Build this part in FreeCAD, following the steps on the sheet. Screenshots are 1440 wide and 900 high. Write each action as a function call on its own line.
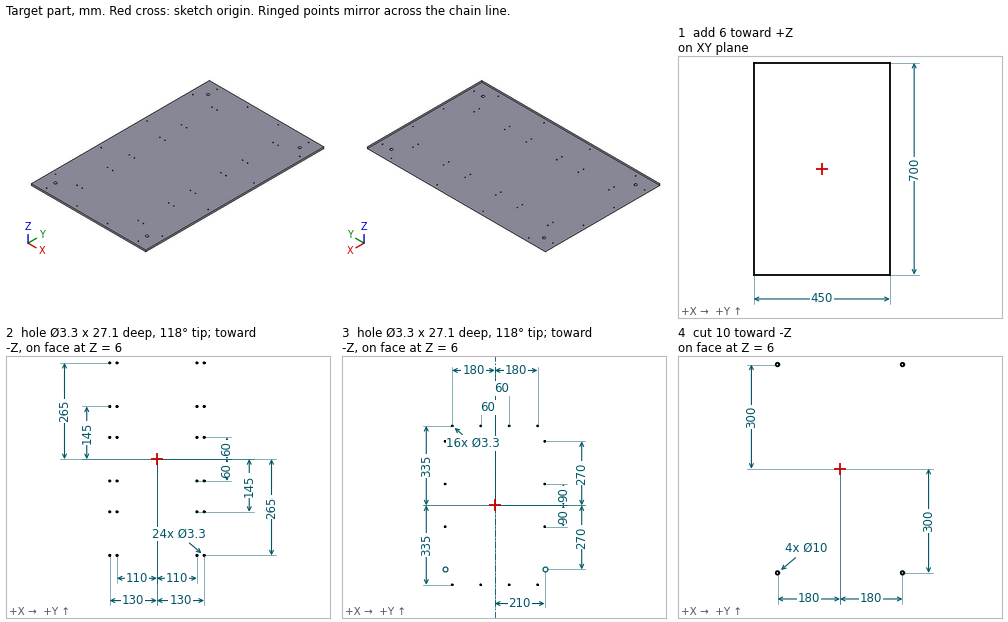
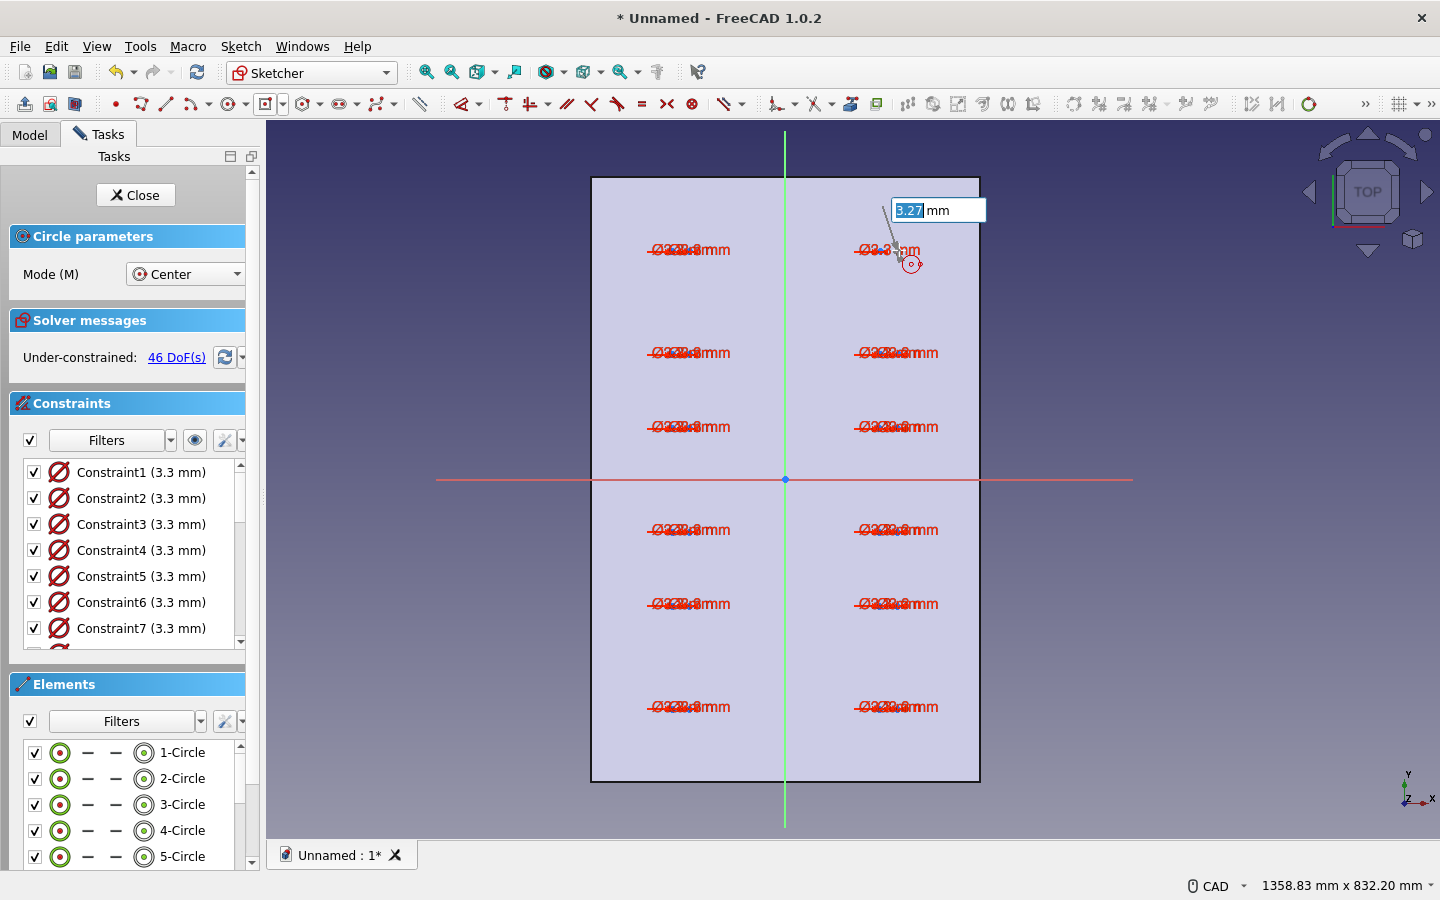
text(3.3)
key(Return)
key(Escape)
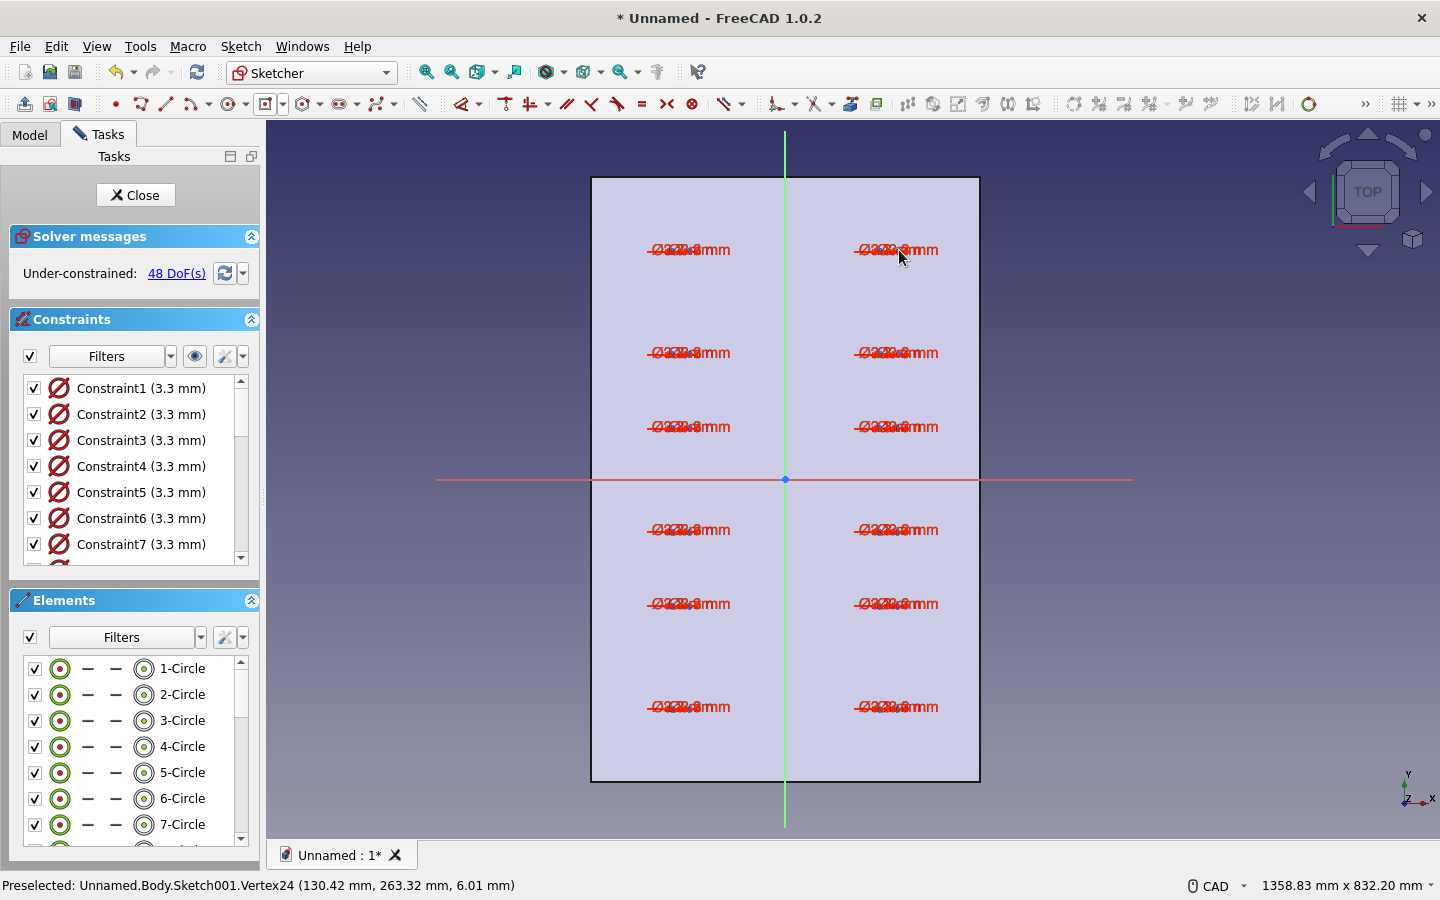
click(898, 709)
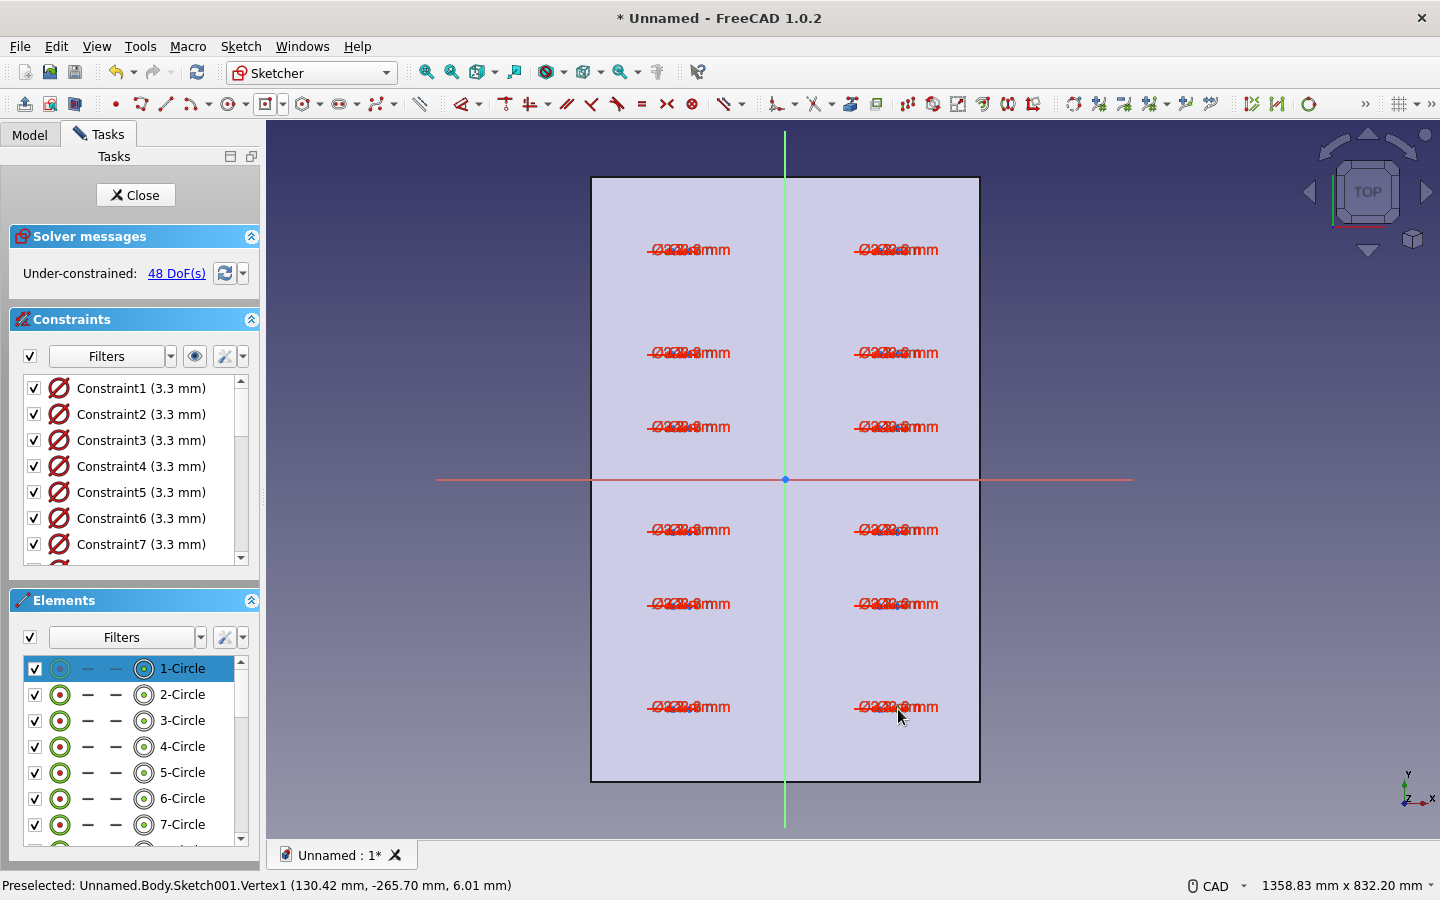
click(880, 709)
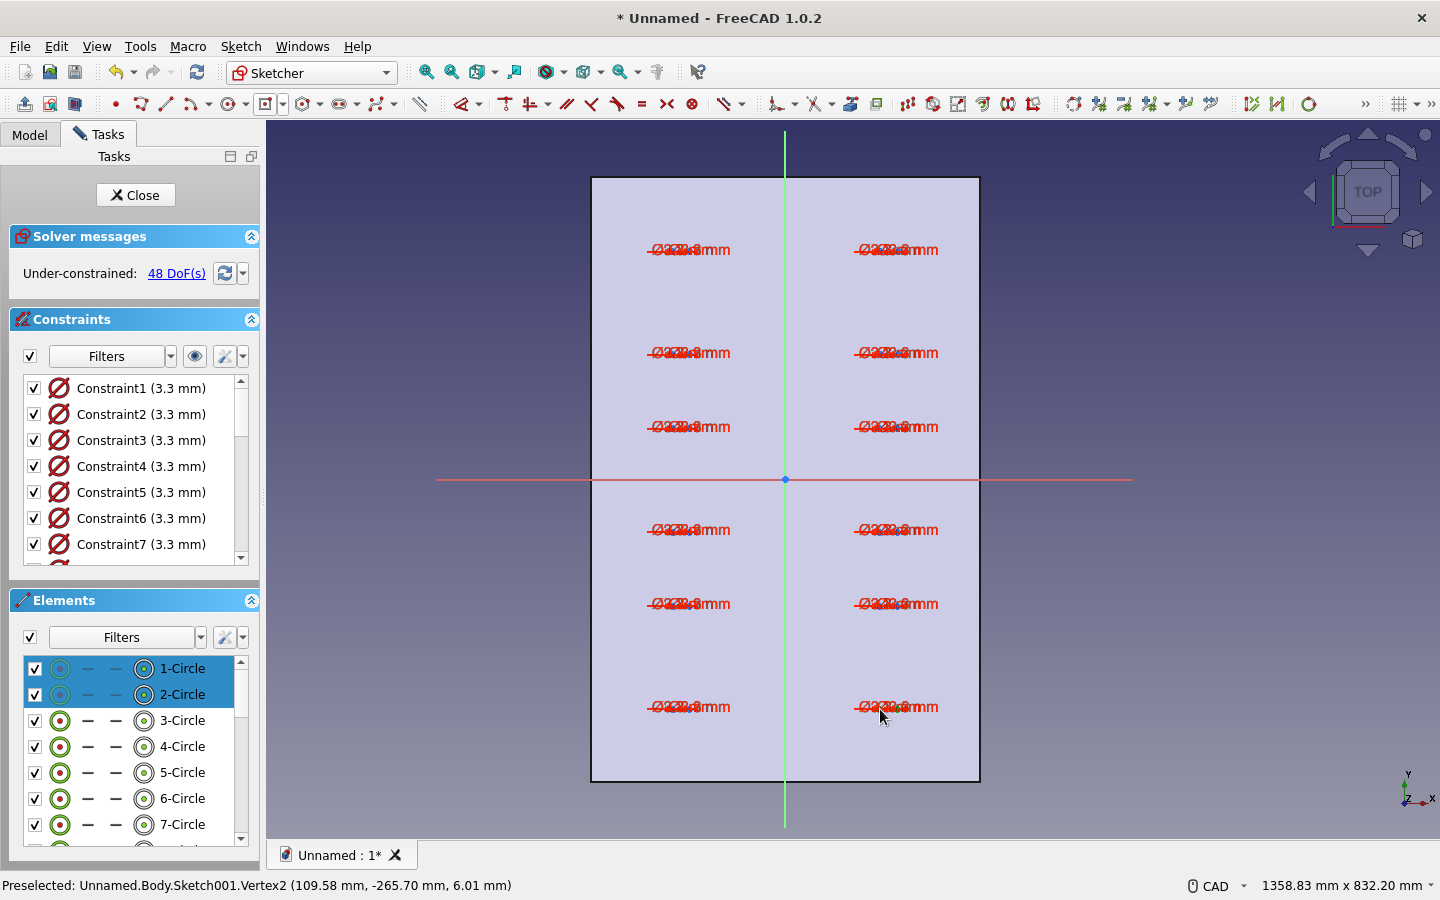
click(548, 104)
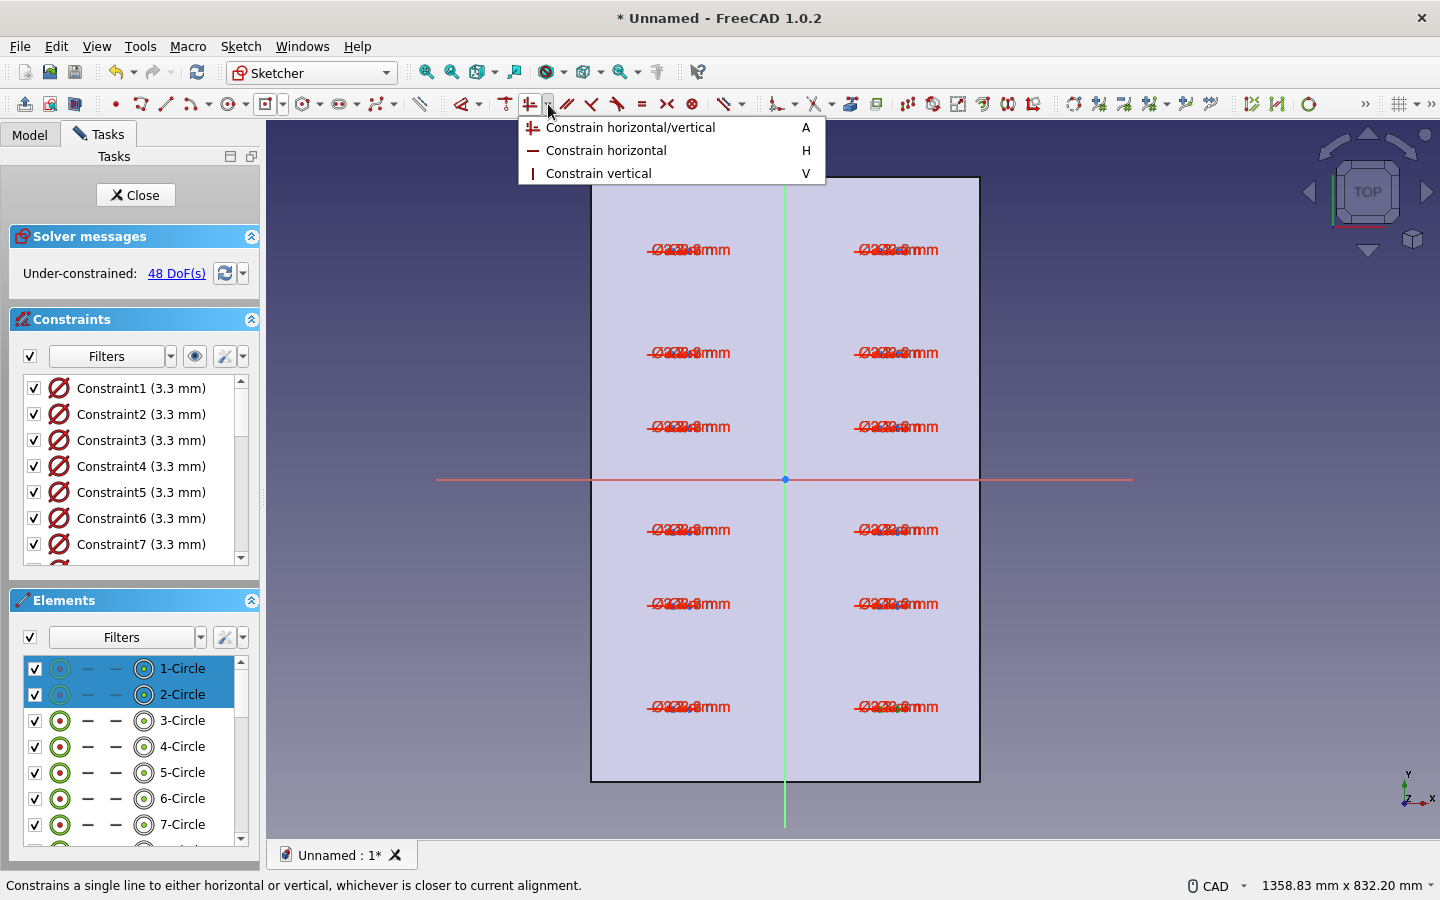
click(672, 150)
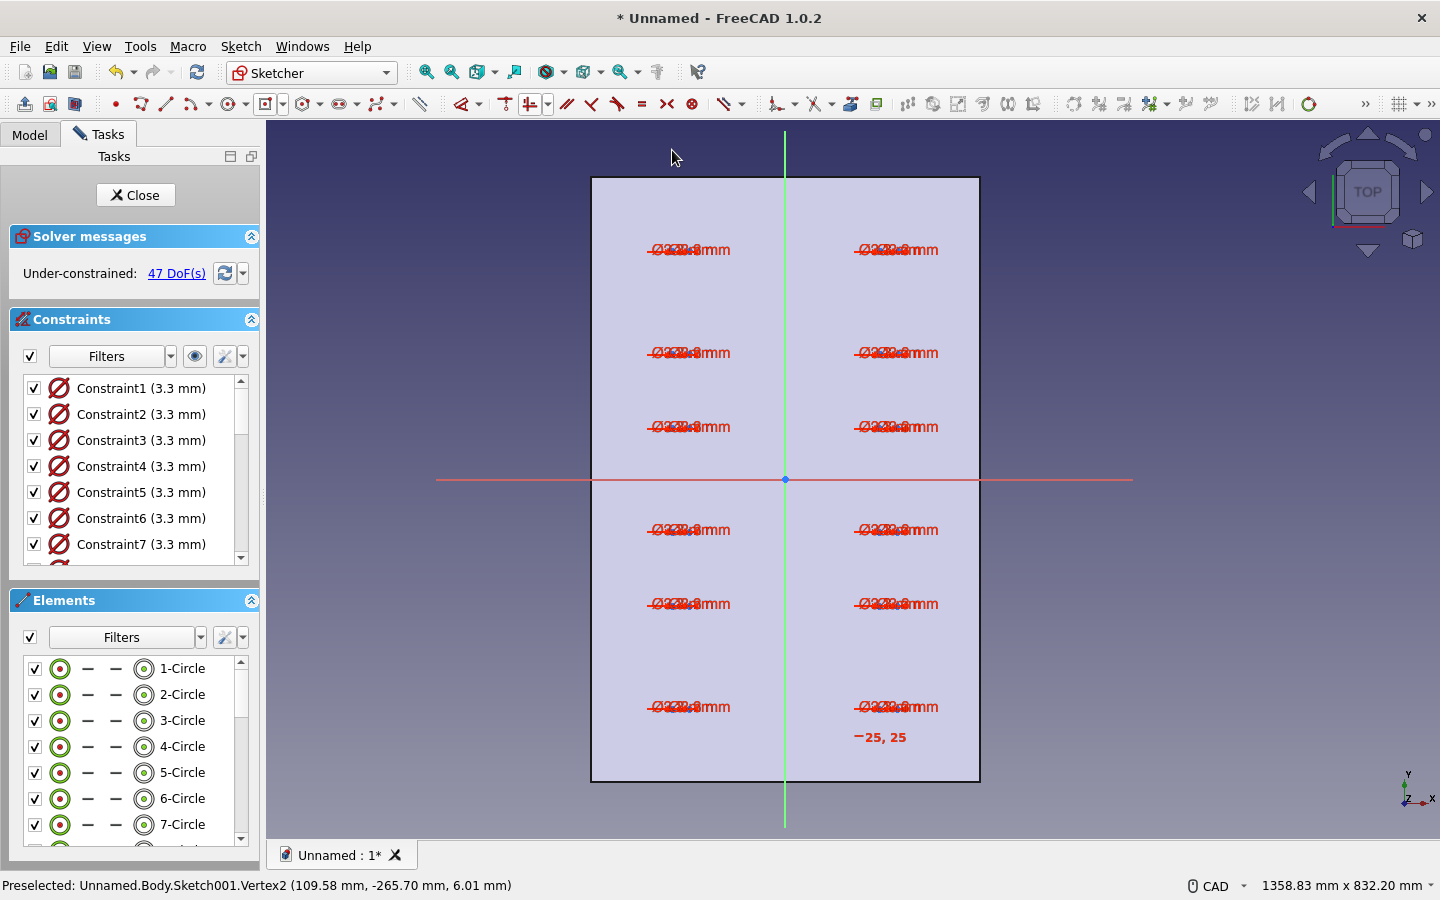
click(880, 709)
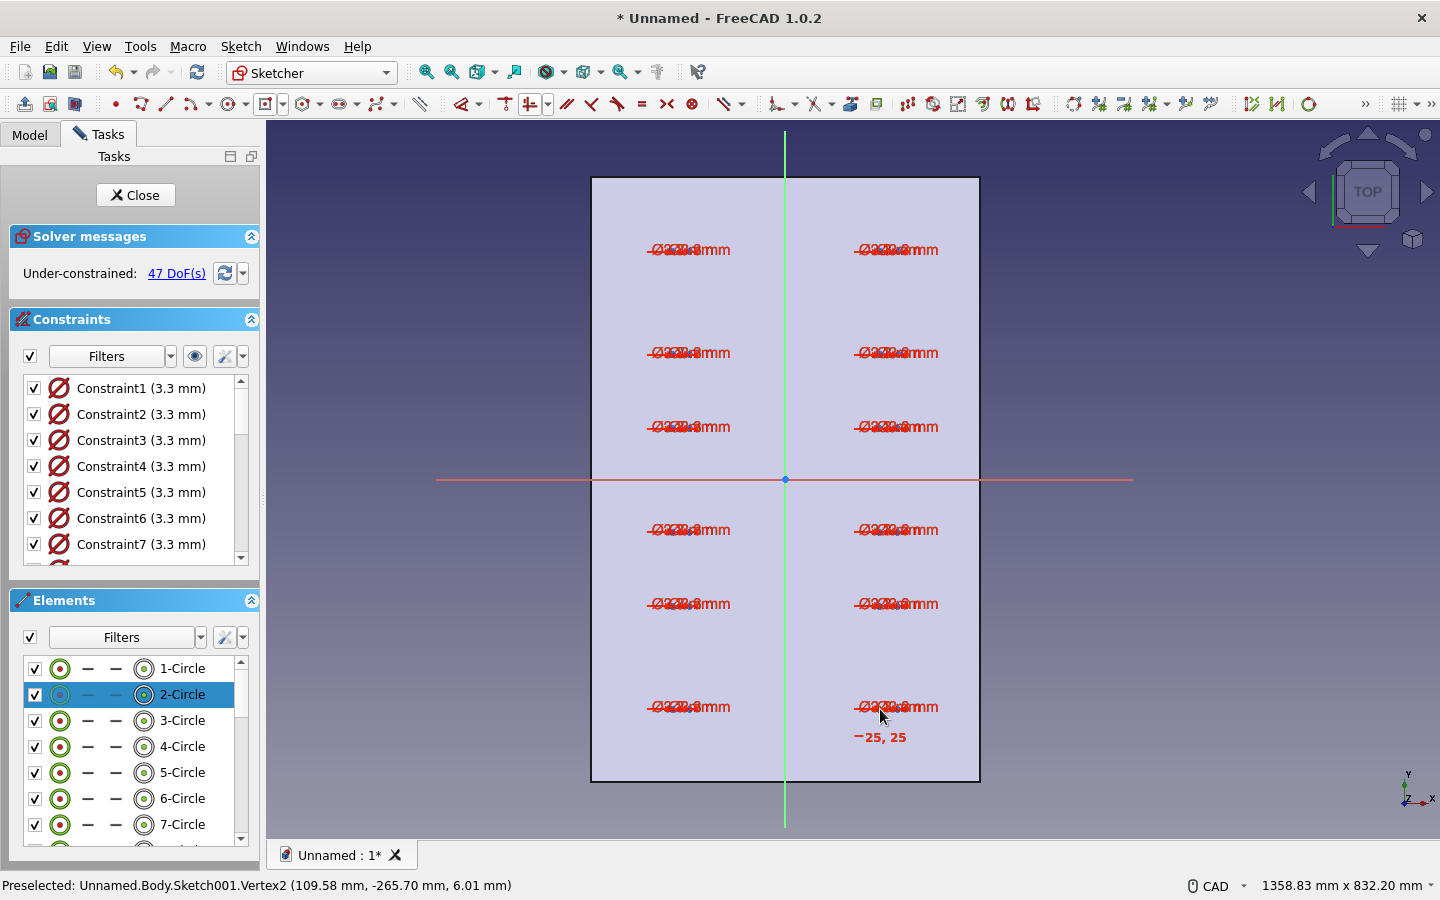
click(880, 606)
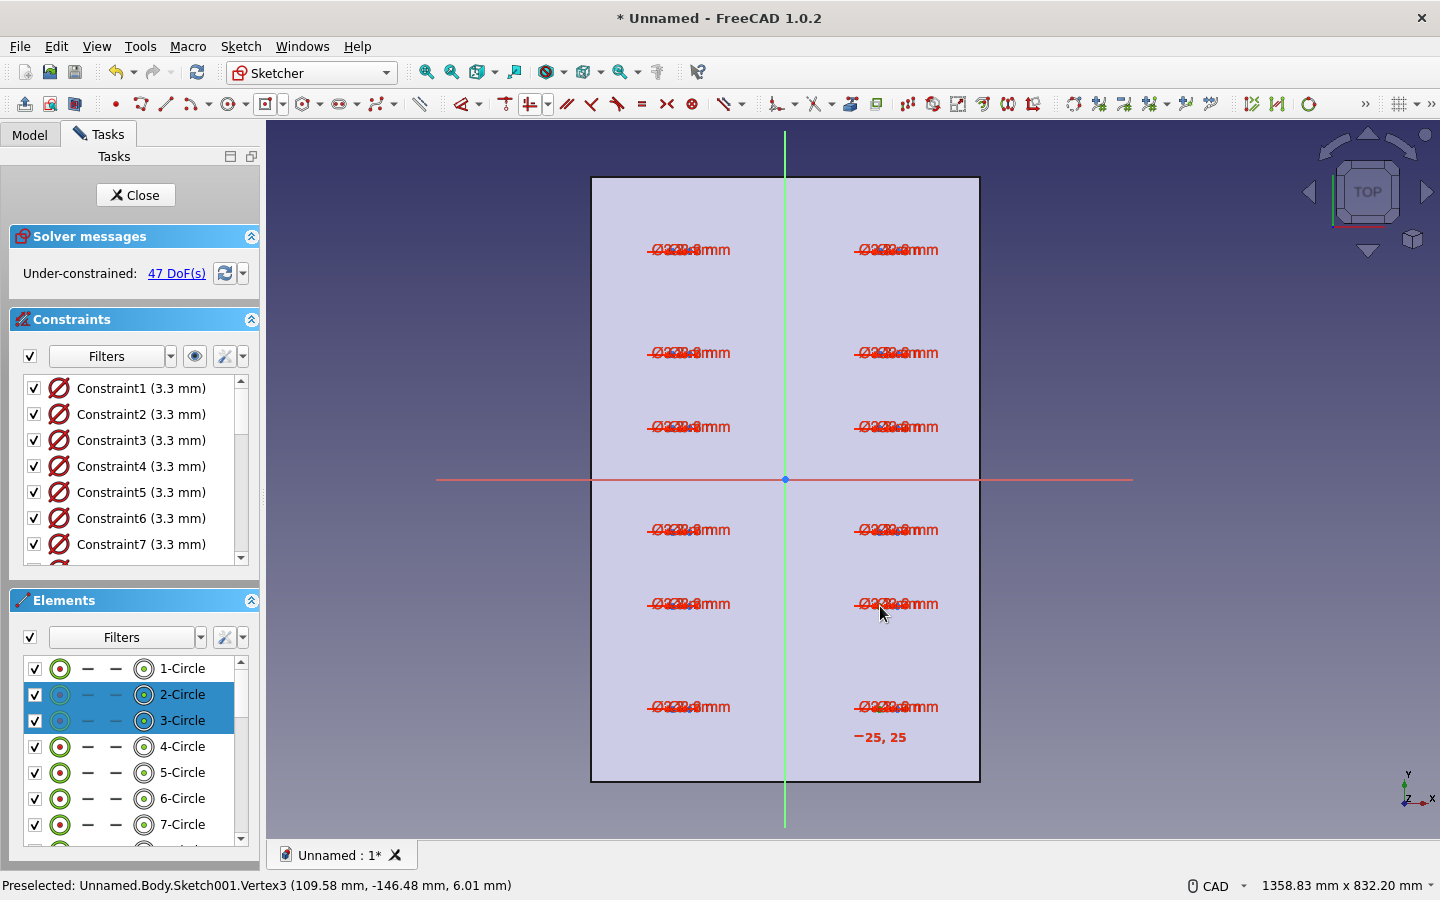
click(548, 104)